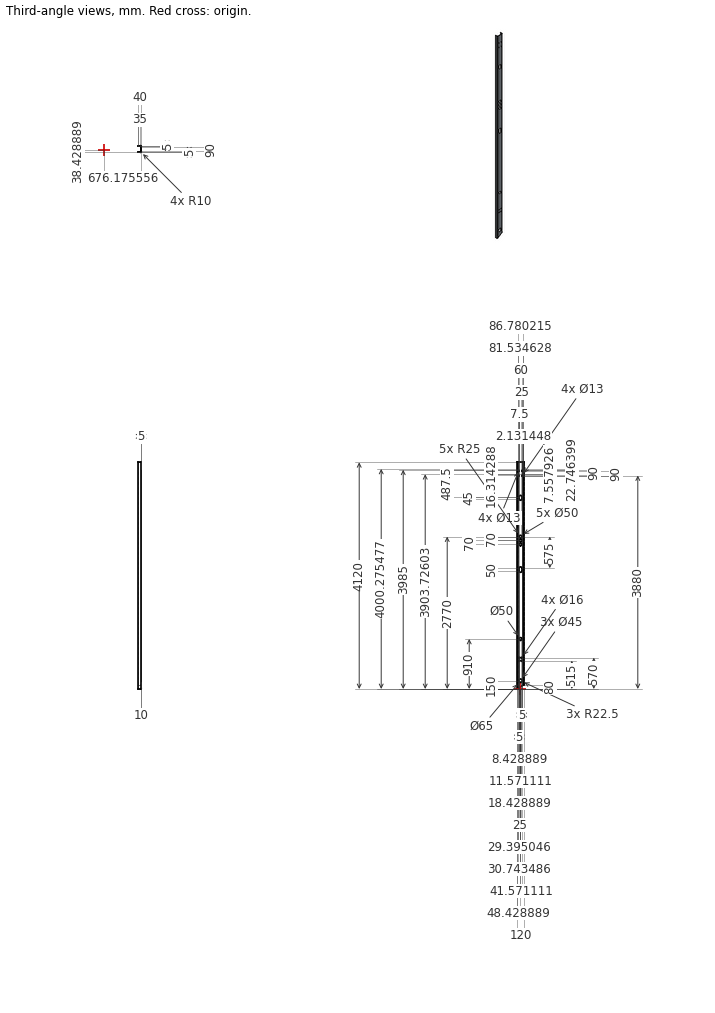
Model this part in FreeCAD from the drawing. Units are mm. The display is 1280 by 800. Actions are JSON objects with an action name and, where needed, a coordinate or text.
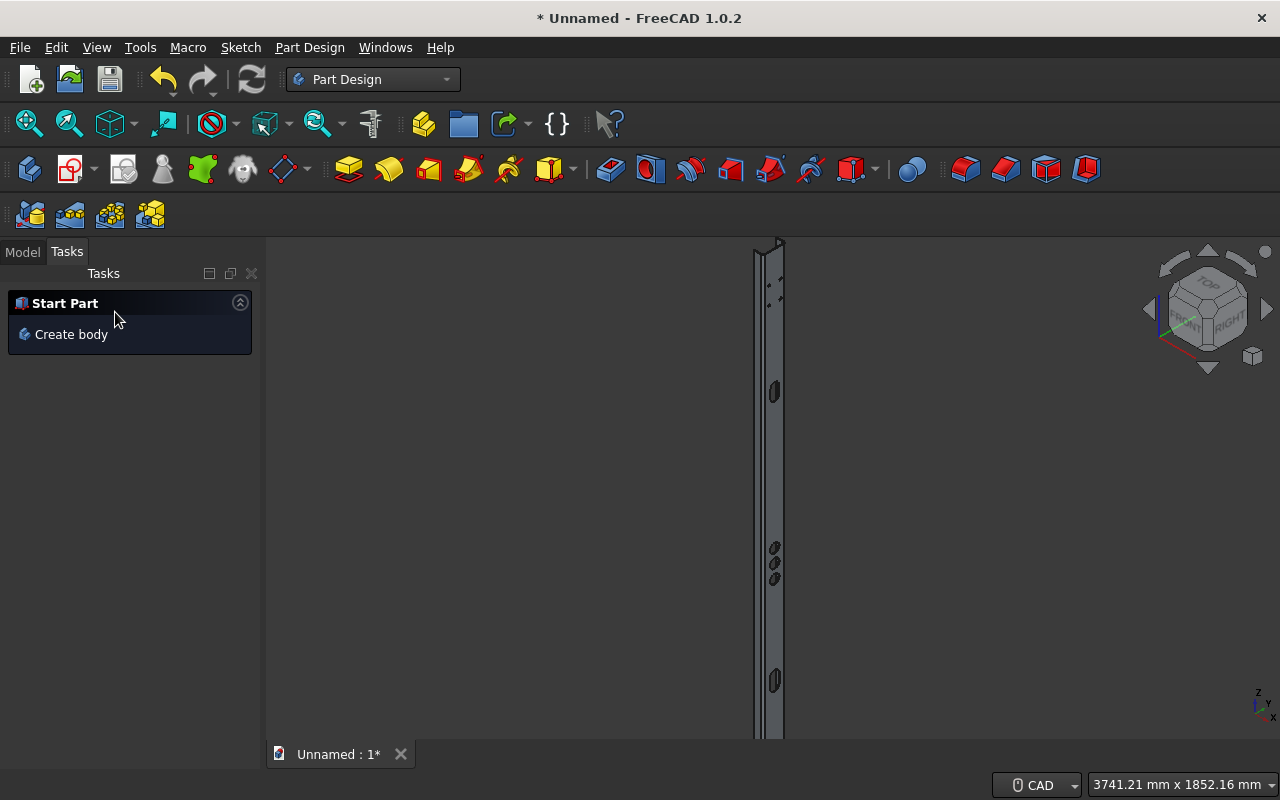
{"action": "key", "text": "v f"}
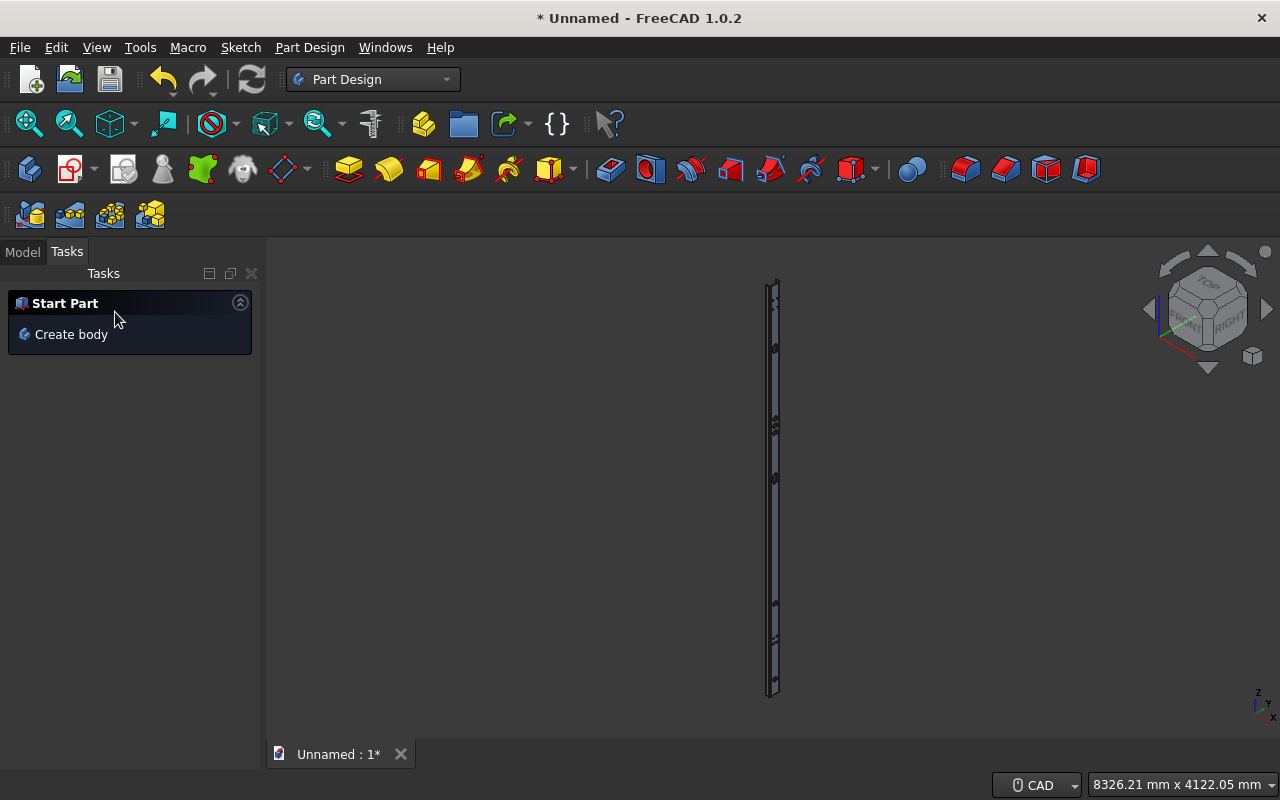
{"action": "scroll", "coordinate": [775, 313], "scroll_direction": "up", "scroll_amount": 4}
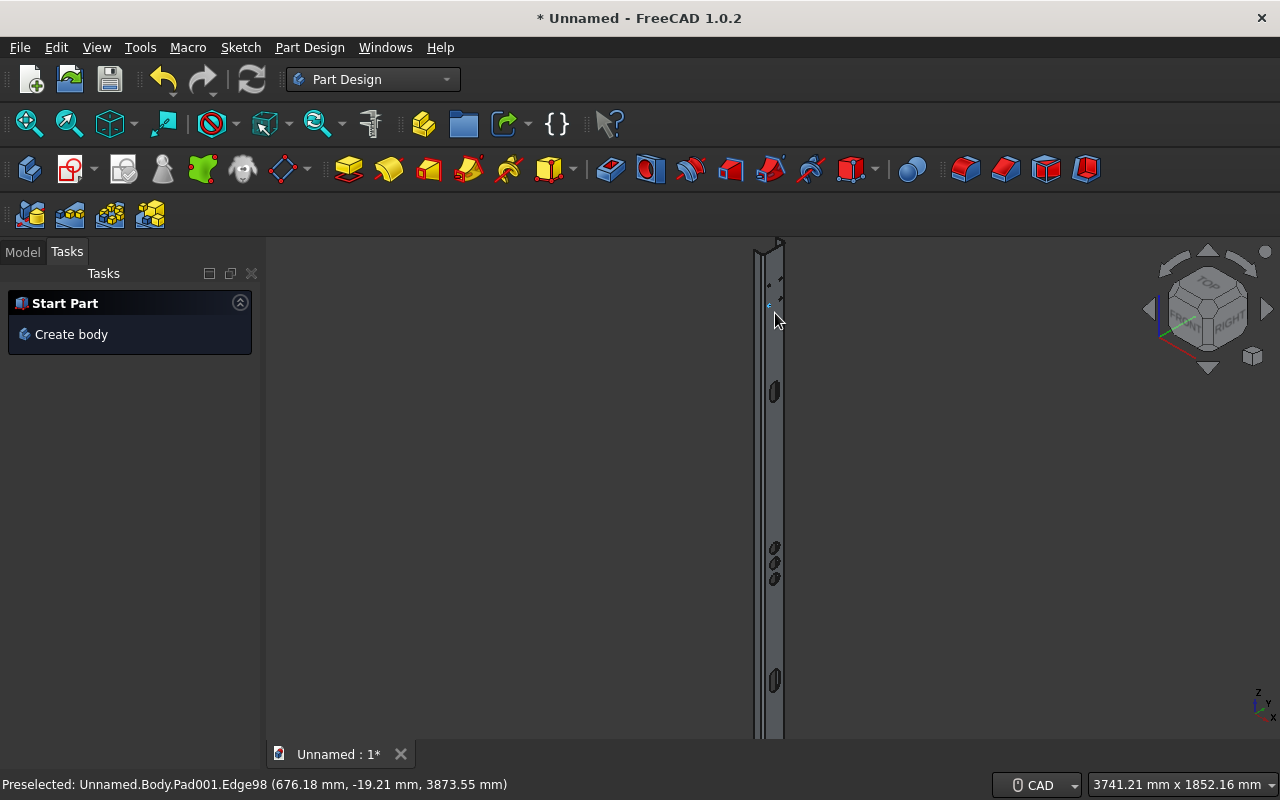
{"action": "left_click", "coordinate": [775, 444]}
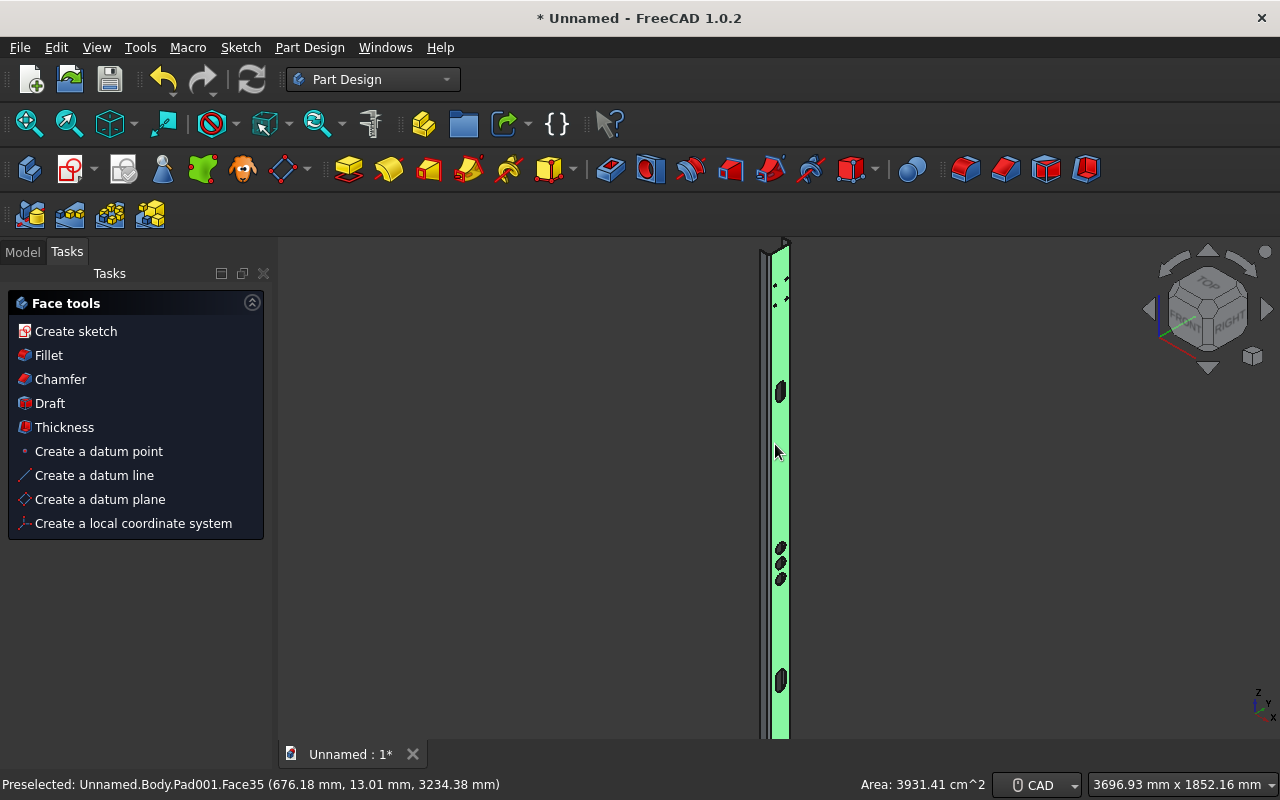
{"action": "left_click", "coordinate": [70, 170]}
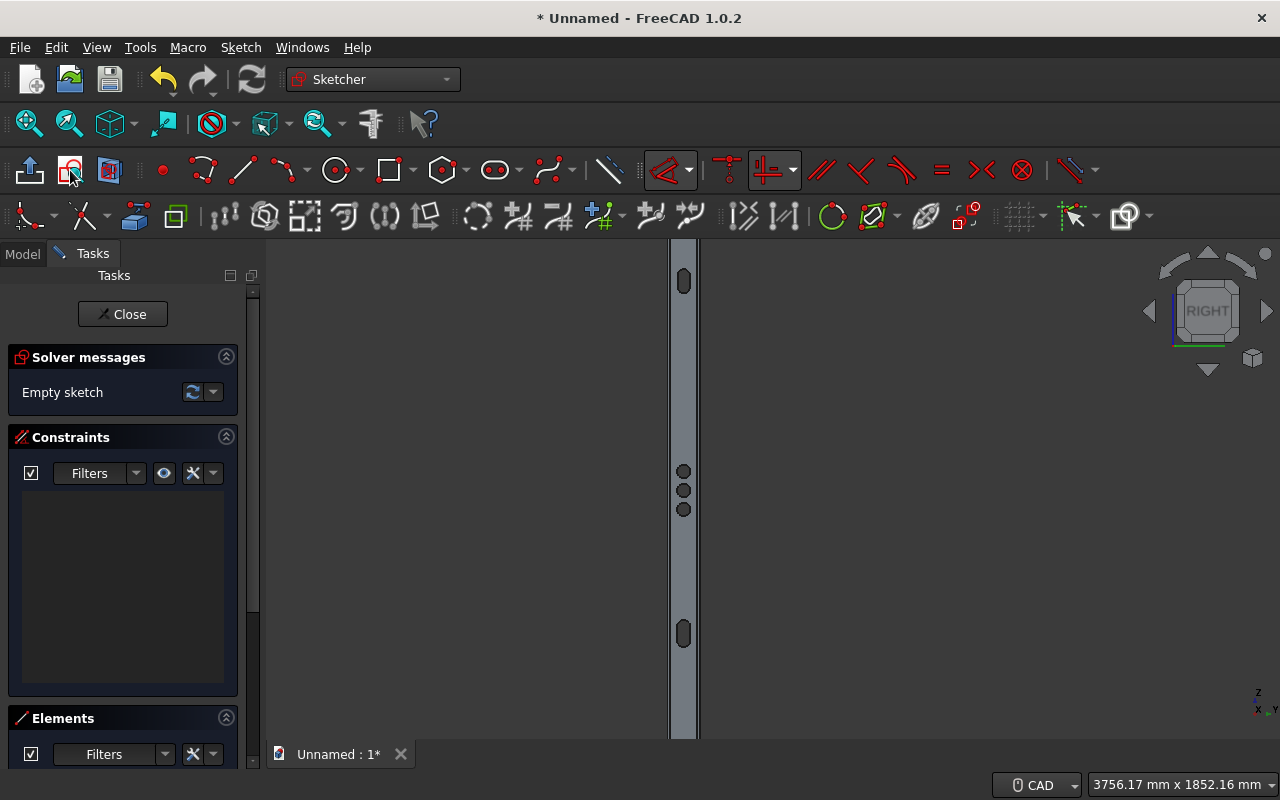
{"action": "scroll", "coordinate": [704, 489], "scroll_direction": "down", "scroll_amount": 5}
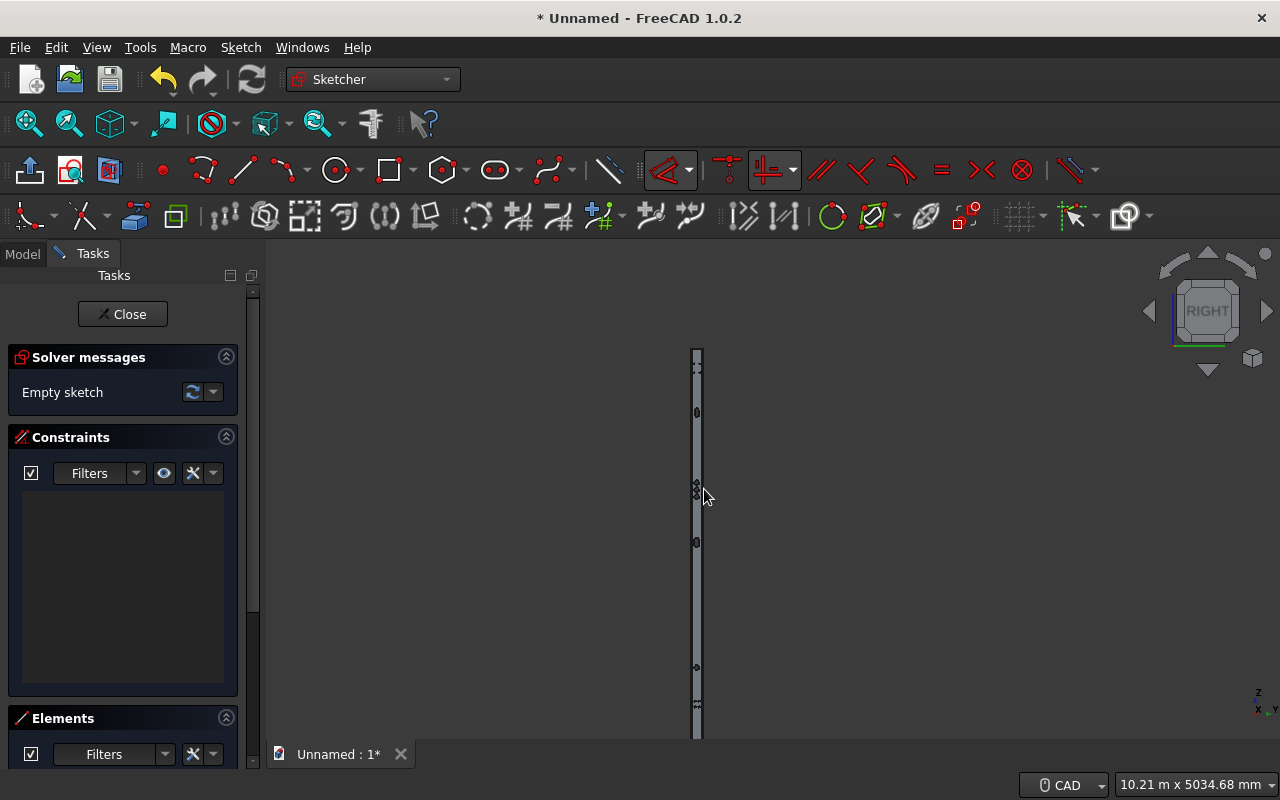
{"action": "scroll", "coordinate": [704, 489], "scroll_direction": "down", "scroll_amount": 5}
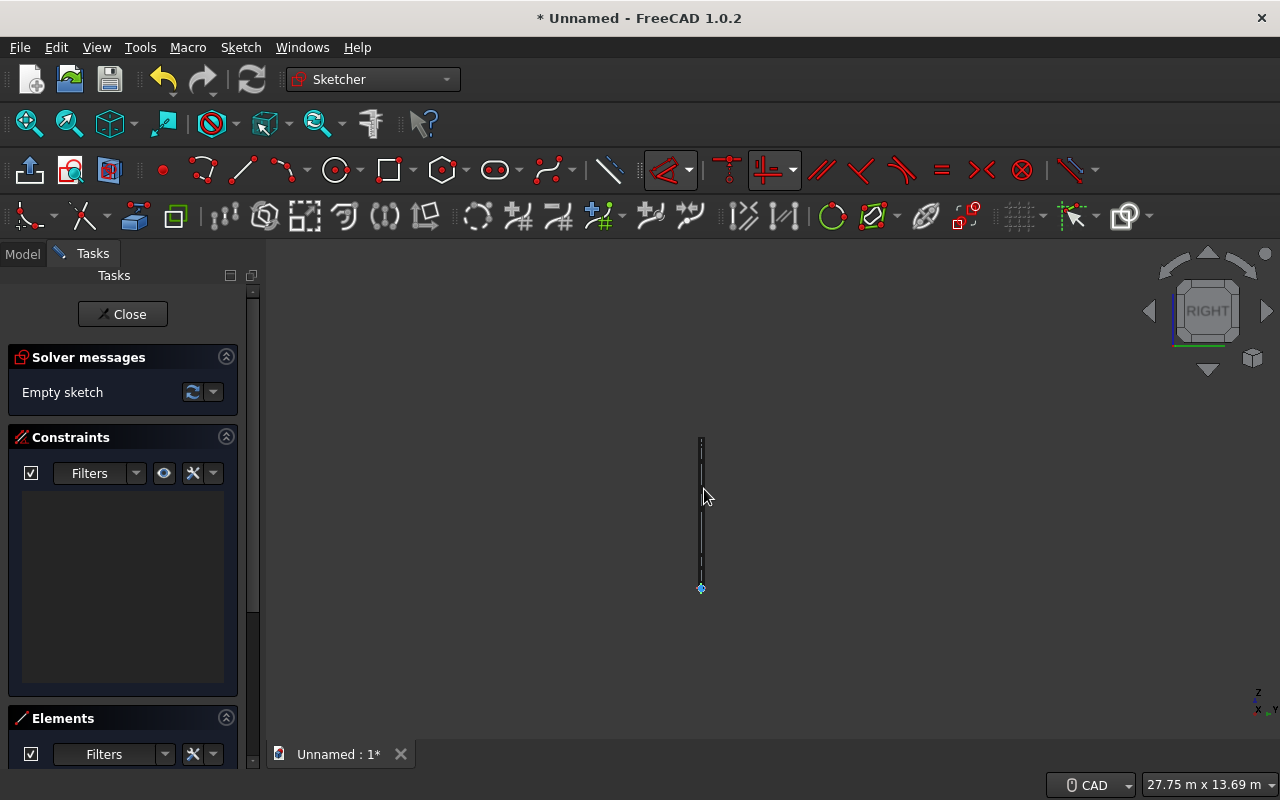
{"action": "scroll", "coordinate": [701, 588], "scroll_direction": "up", "scroll_amount": 15}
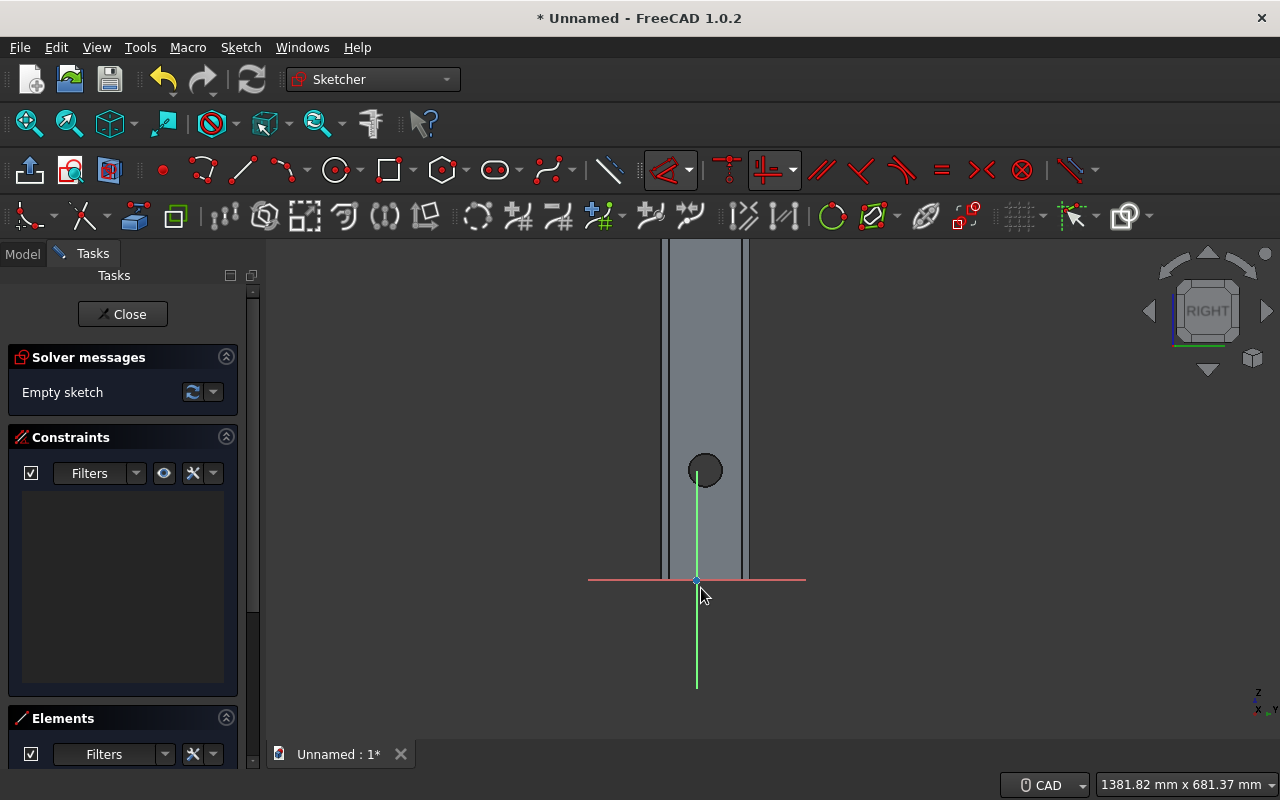
{"action": "scroll", "coordinate": [706, 466], "scroll_direction": "up", "scroll_amount": 9}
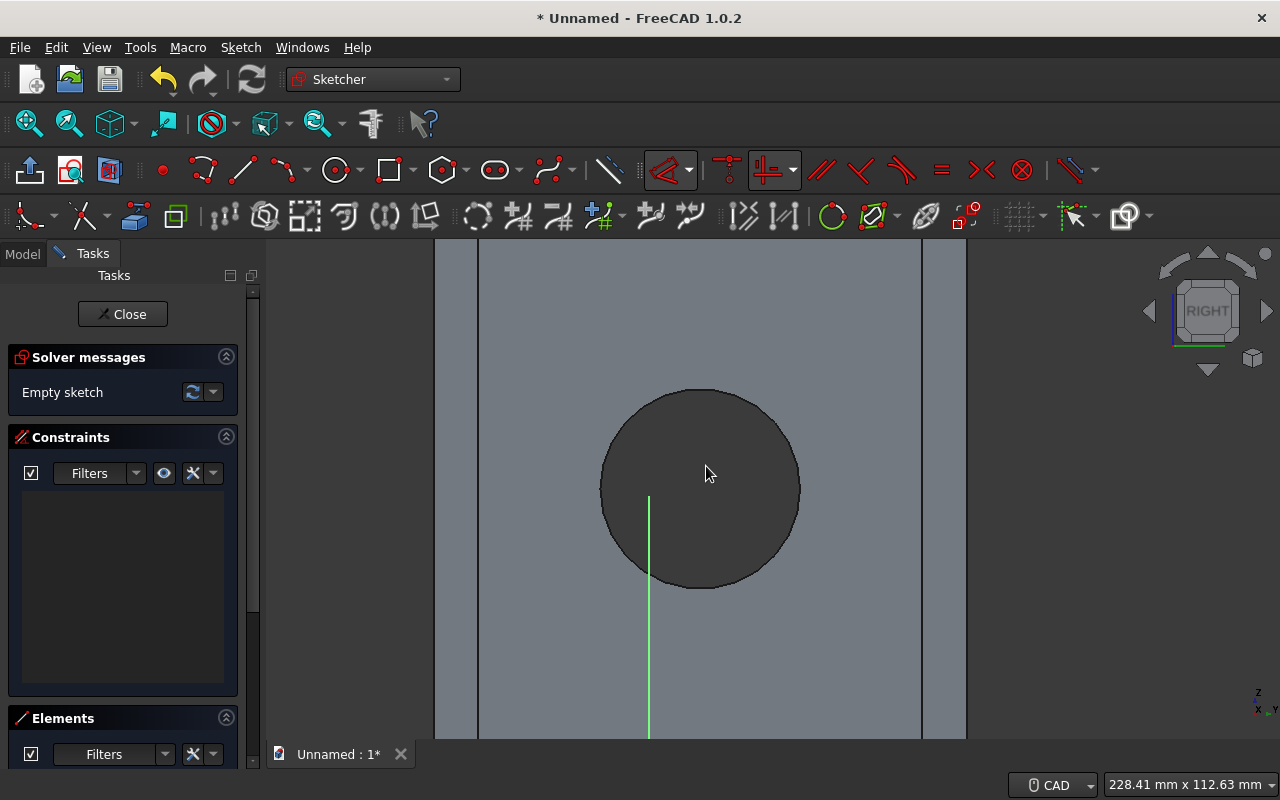
{"action": "key", "text": "g c"}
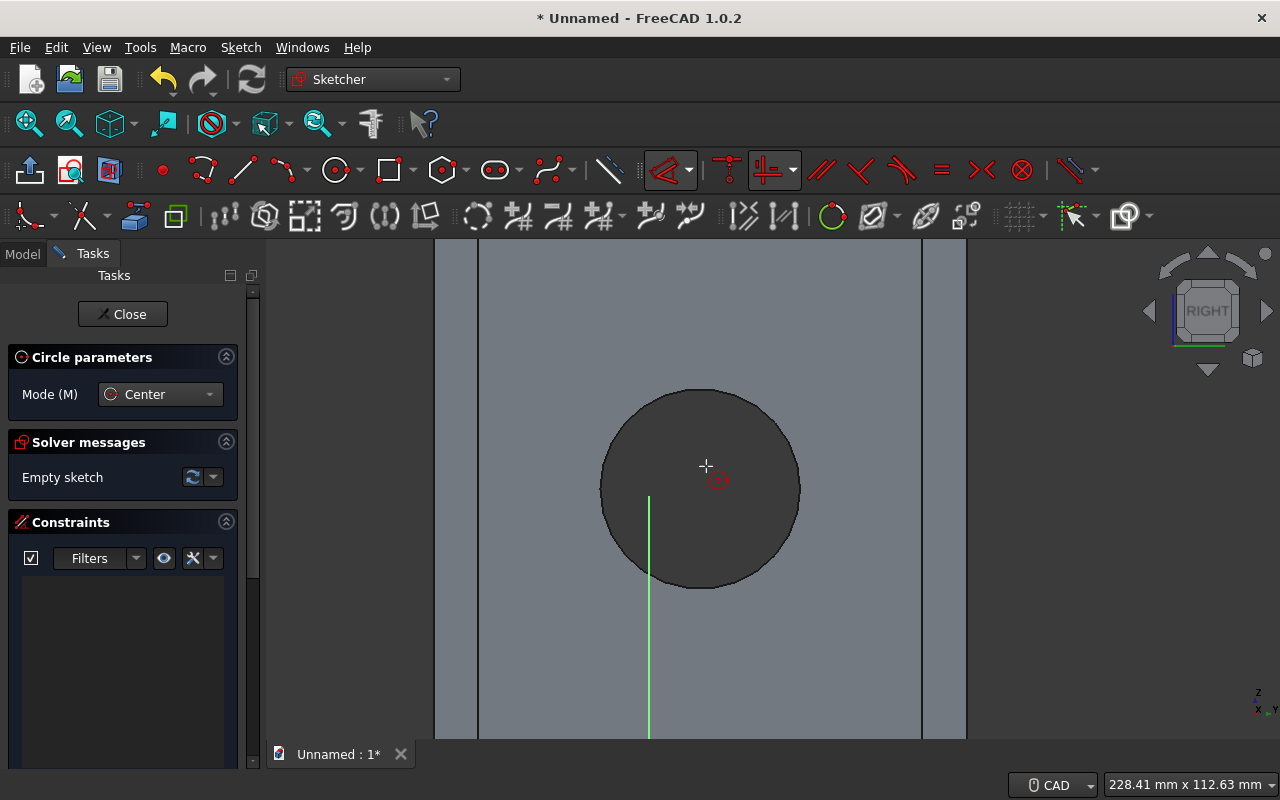
{"action": "left_click", "coordinate": [700, 489]}
{"action": "mouse_move", "coordinate": [802, 387]}